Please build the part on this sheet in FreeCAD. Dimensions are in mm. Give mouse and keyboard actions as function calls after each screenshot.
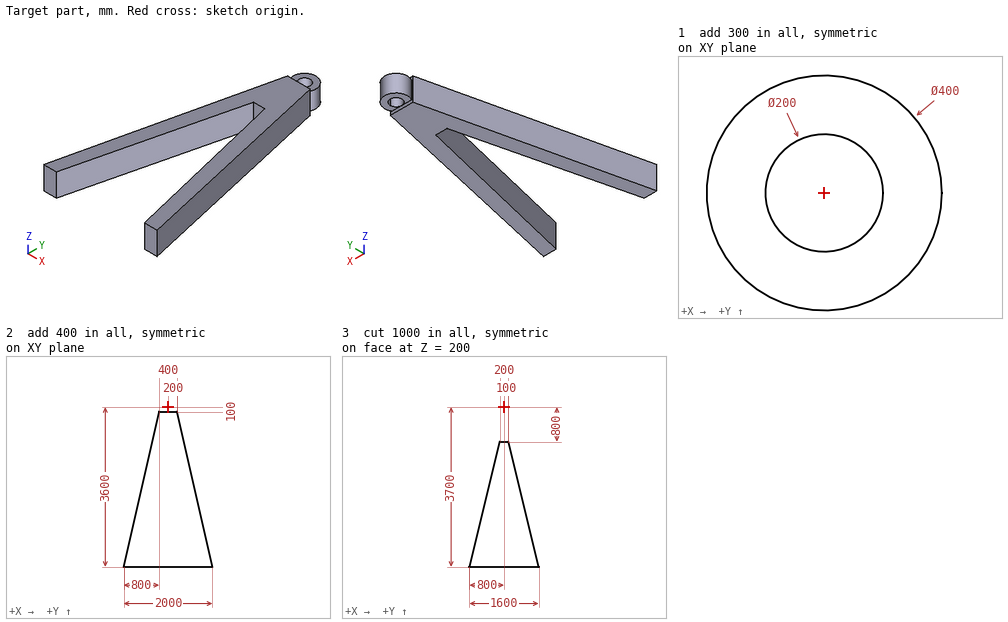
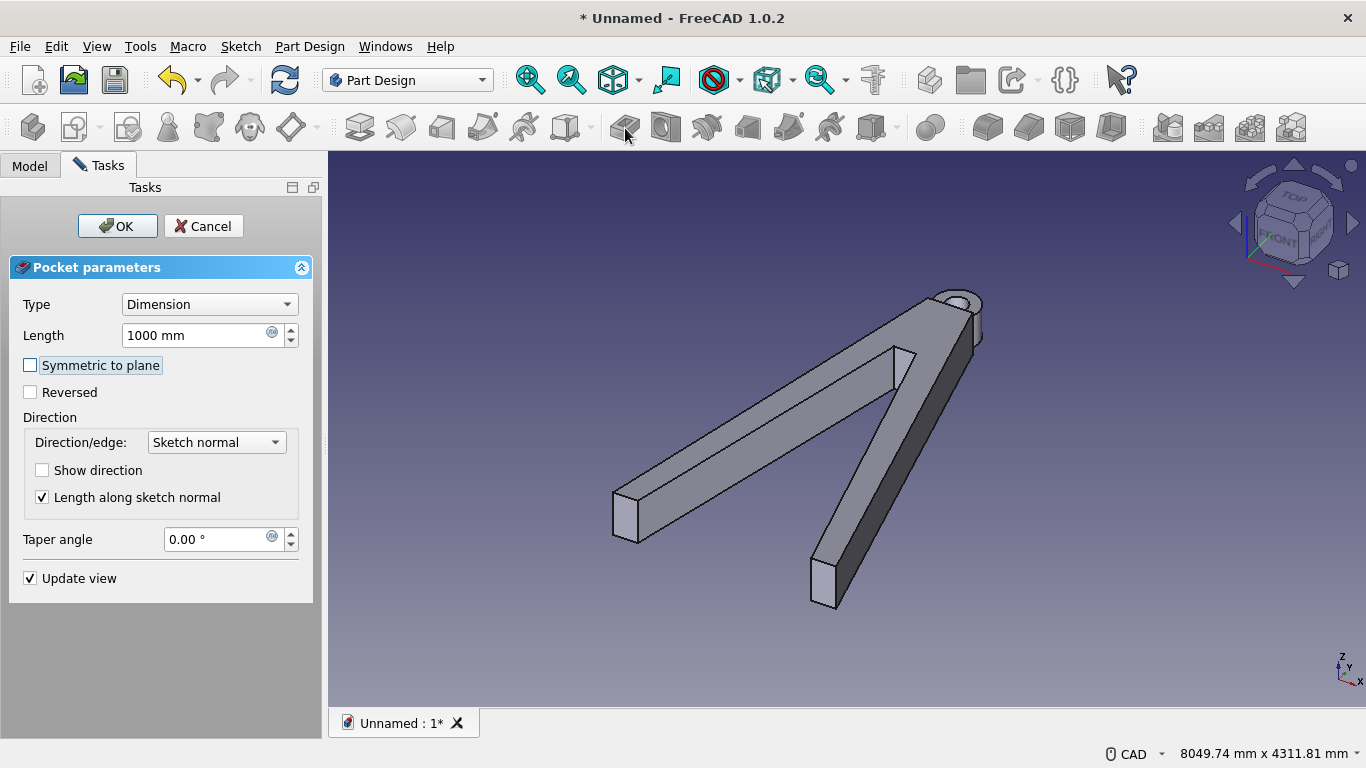
click(31, 365)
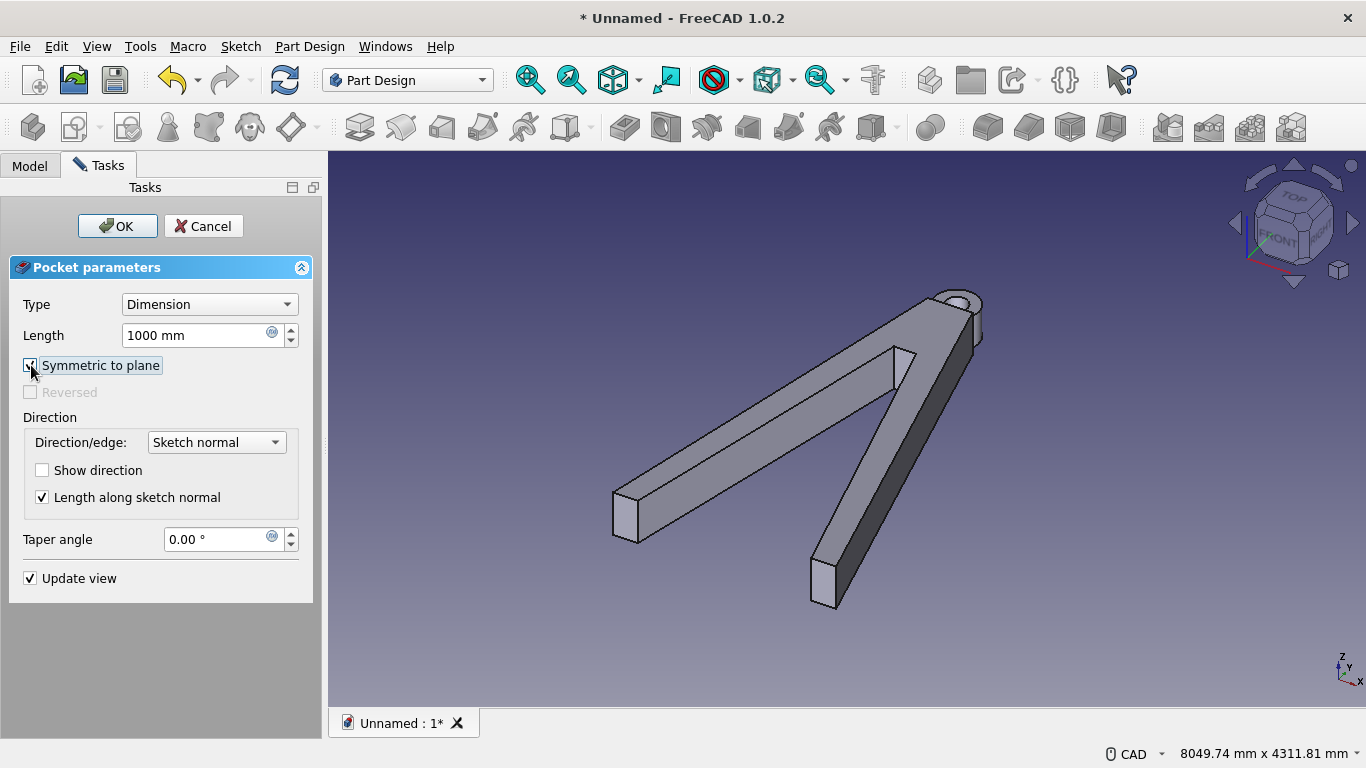
click(118, 226)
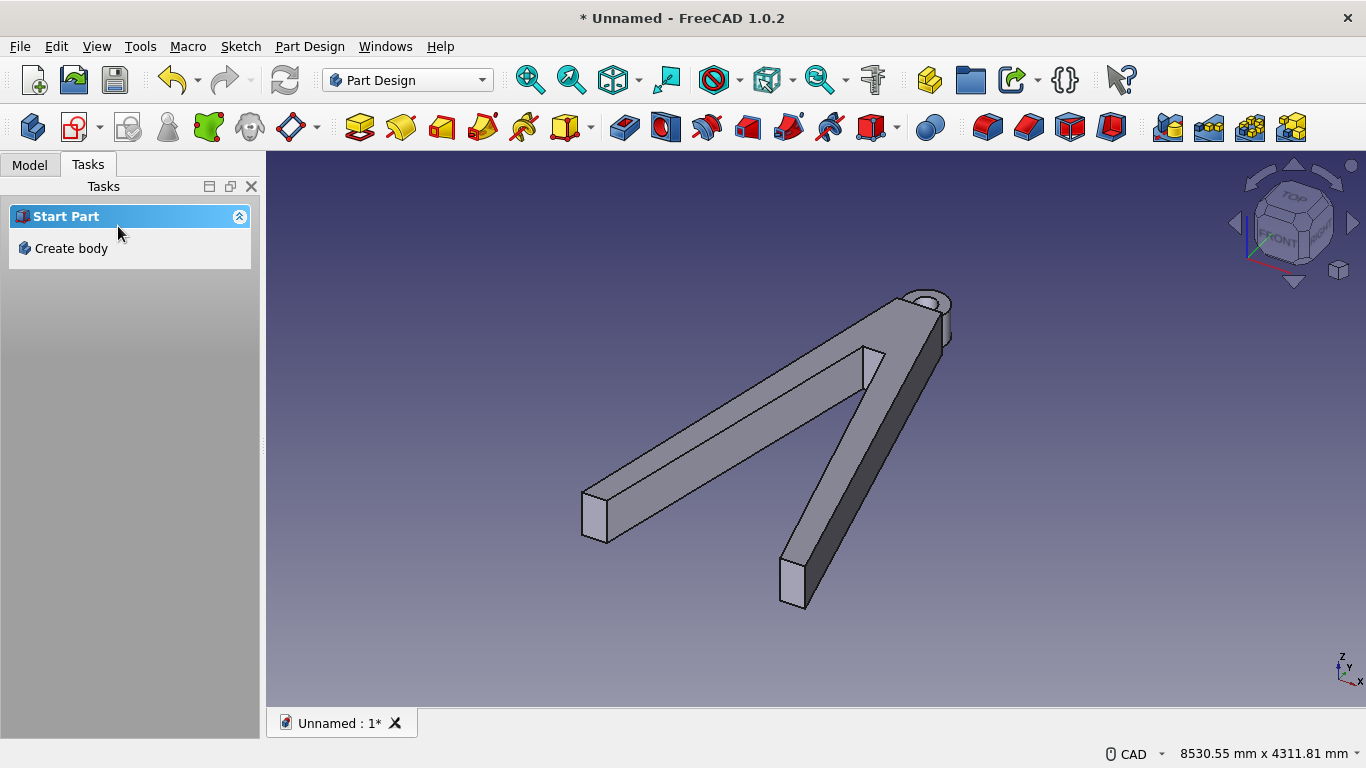
key(0)